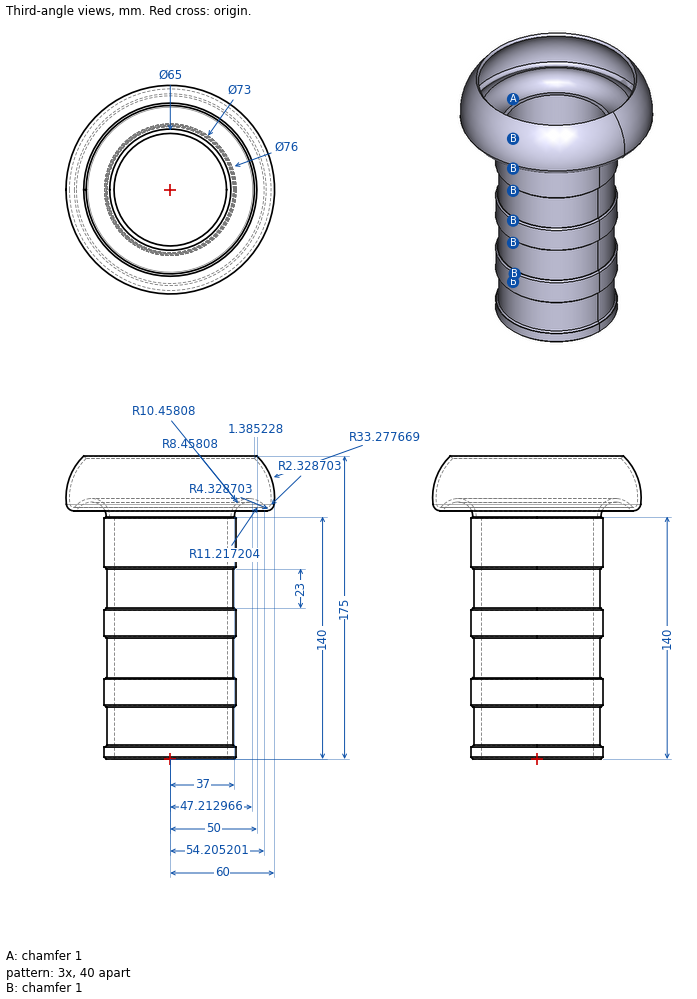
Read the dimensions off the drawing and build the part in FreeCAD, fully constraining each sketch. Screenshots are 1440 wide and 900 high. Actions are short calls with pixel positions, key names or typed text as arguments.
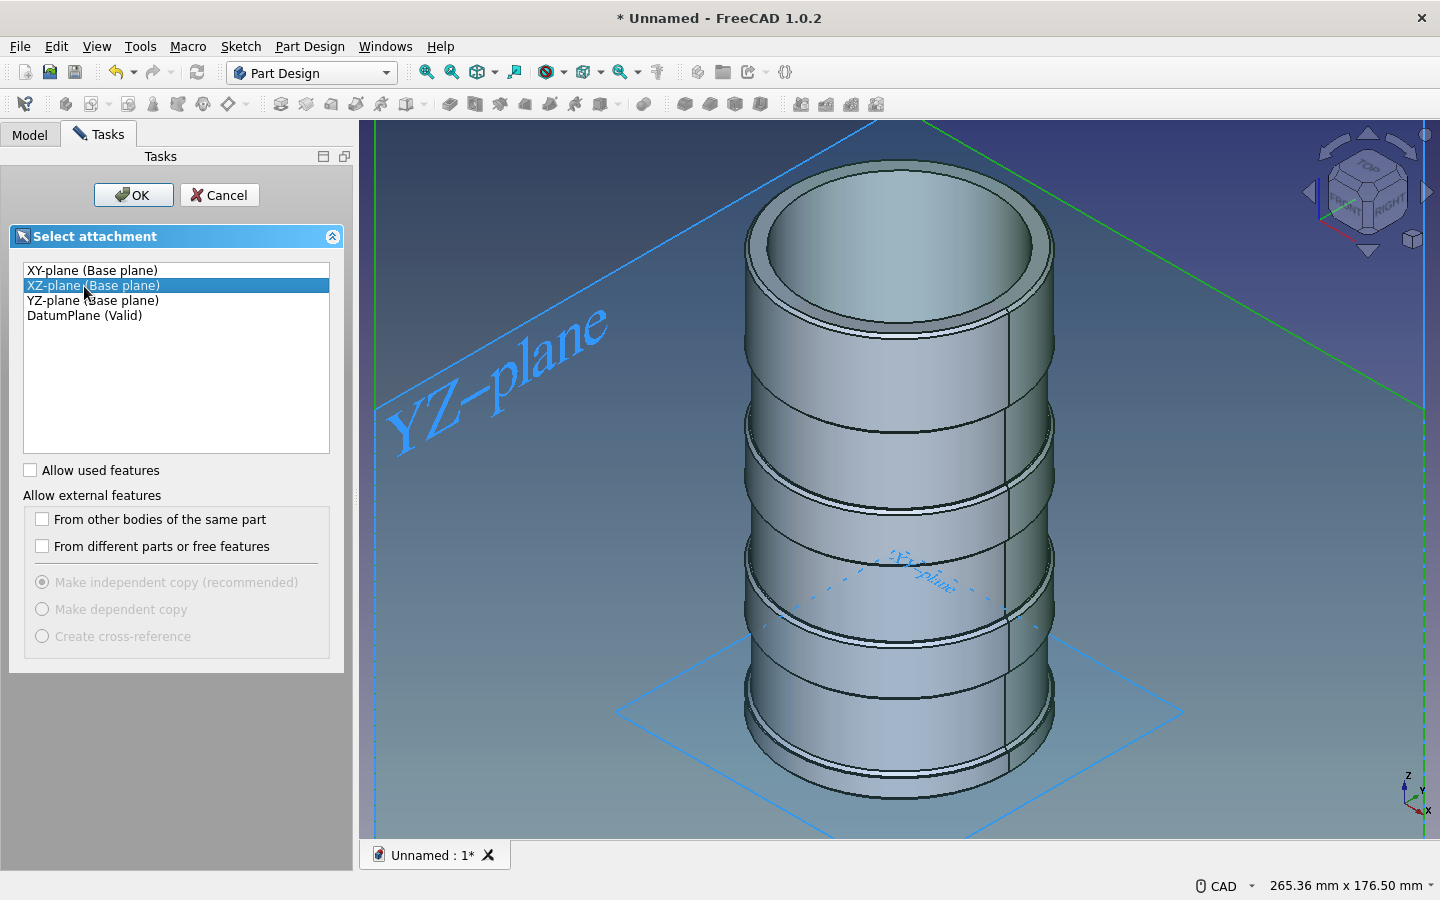
click(134, 195)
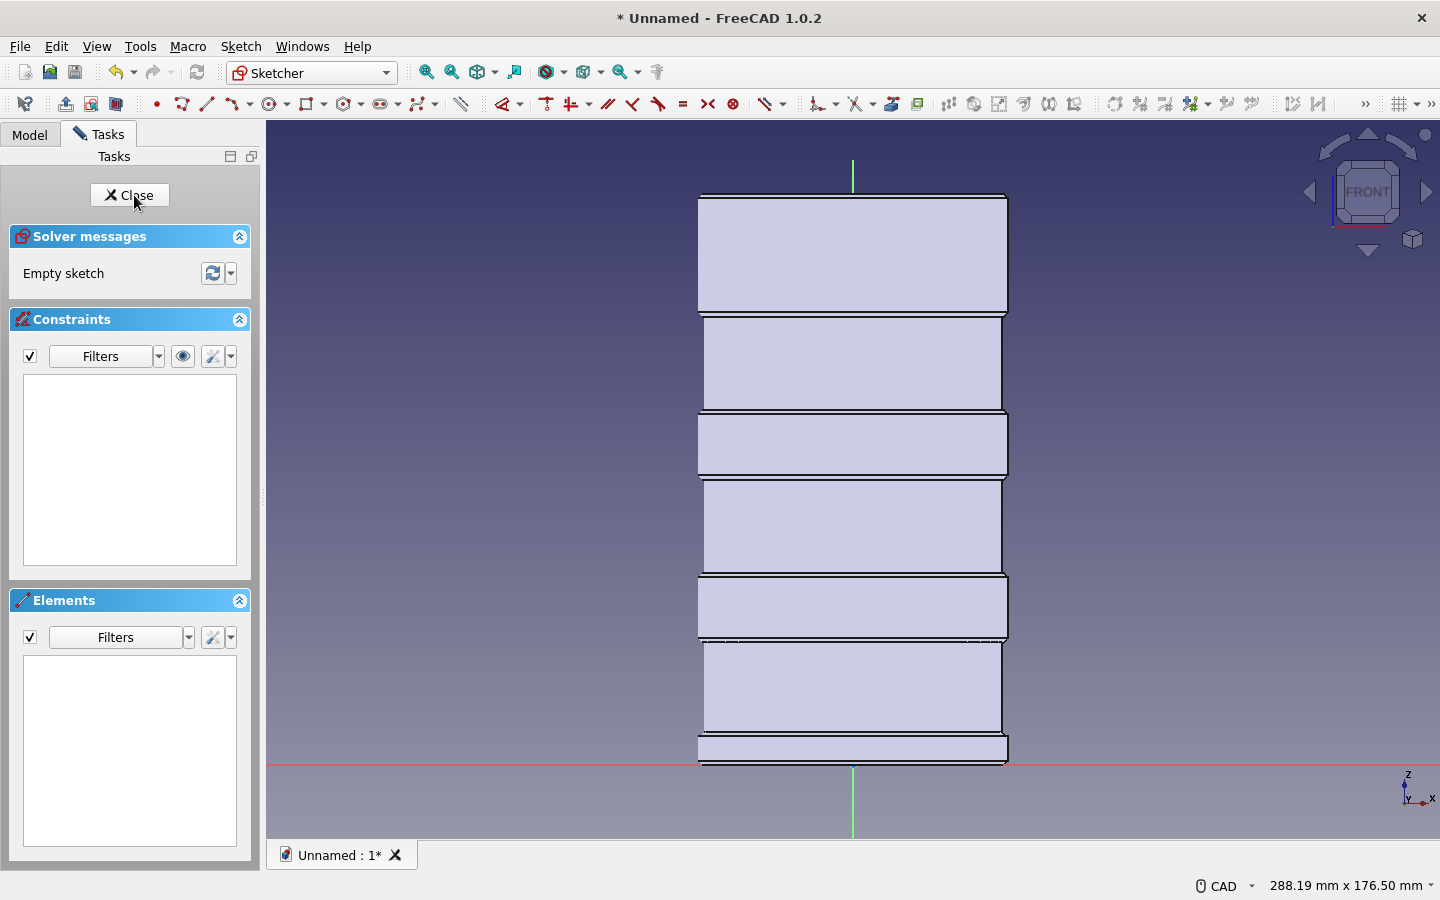
click(116, 104)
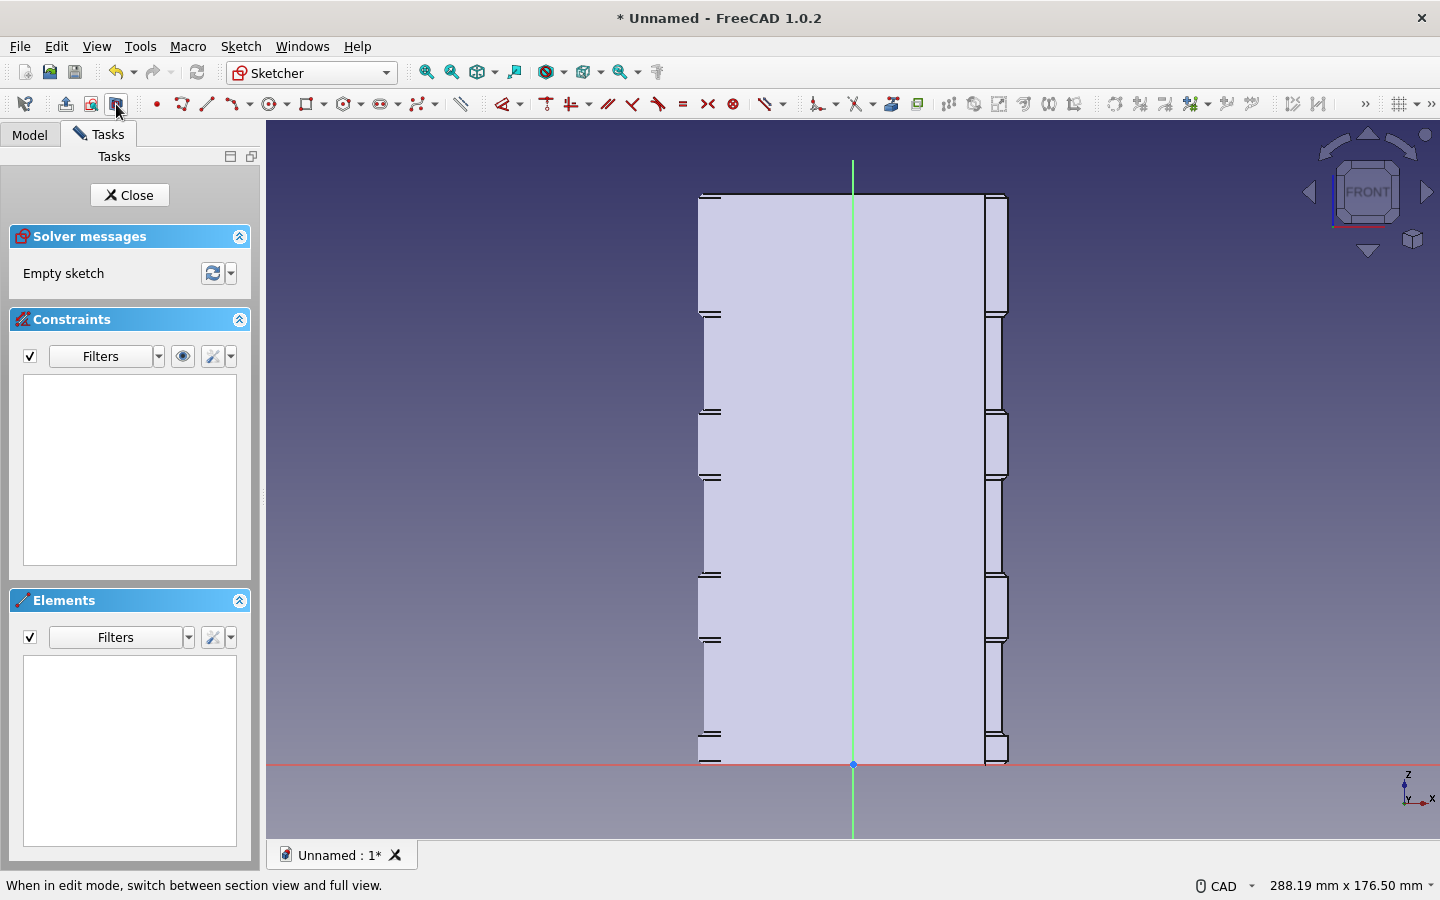
scroll(784, 480, down, 5)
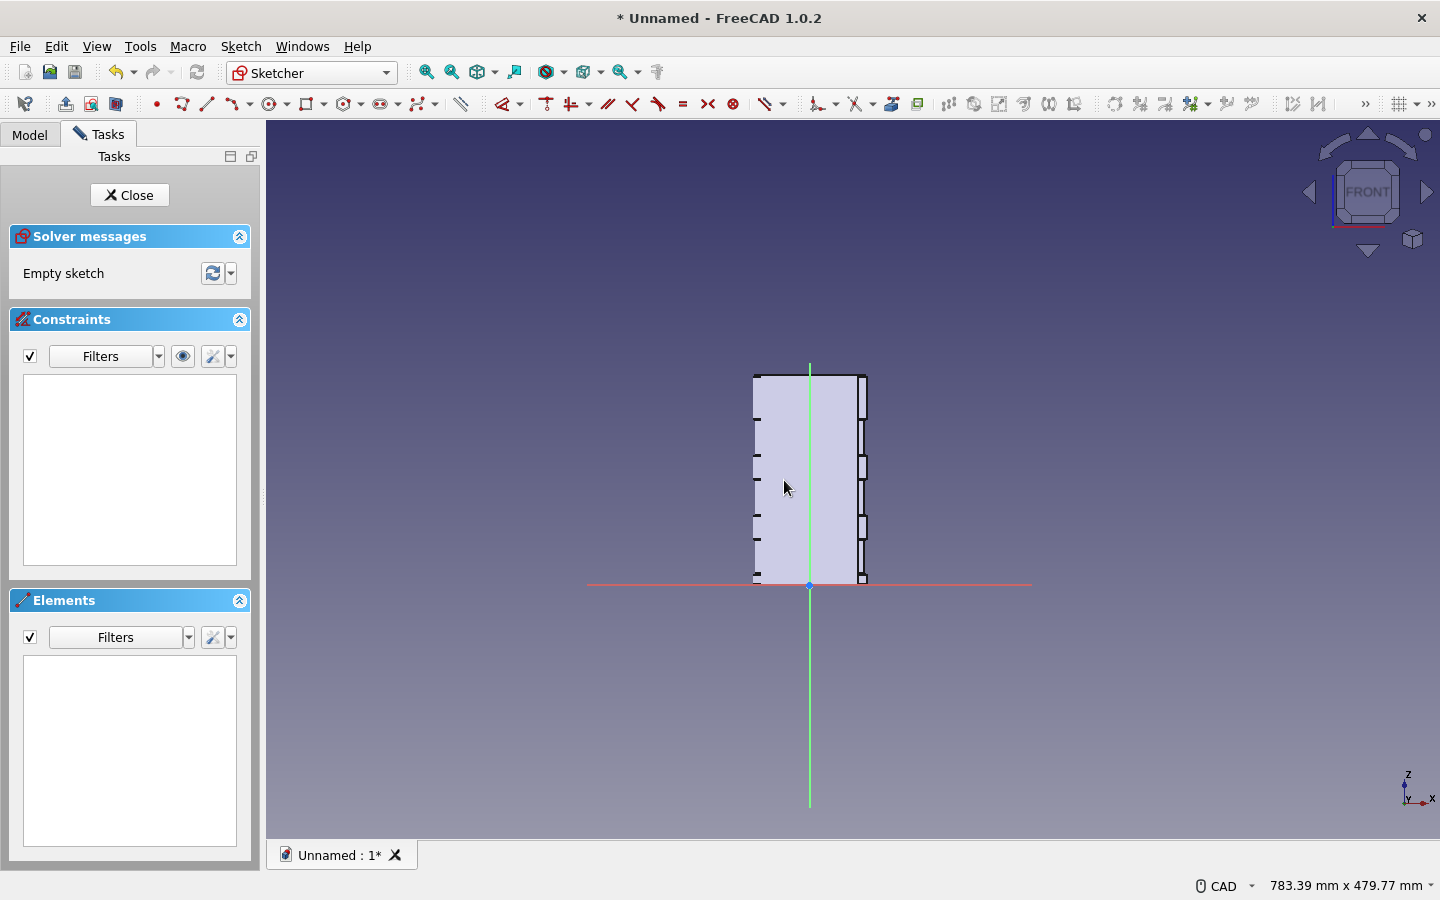
scroll(893, 333, up, 11)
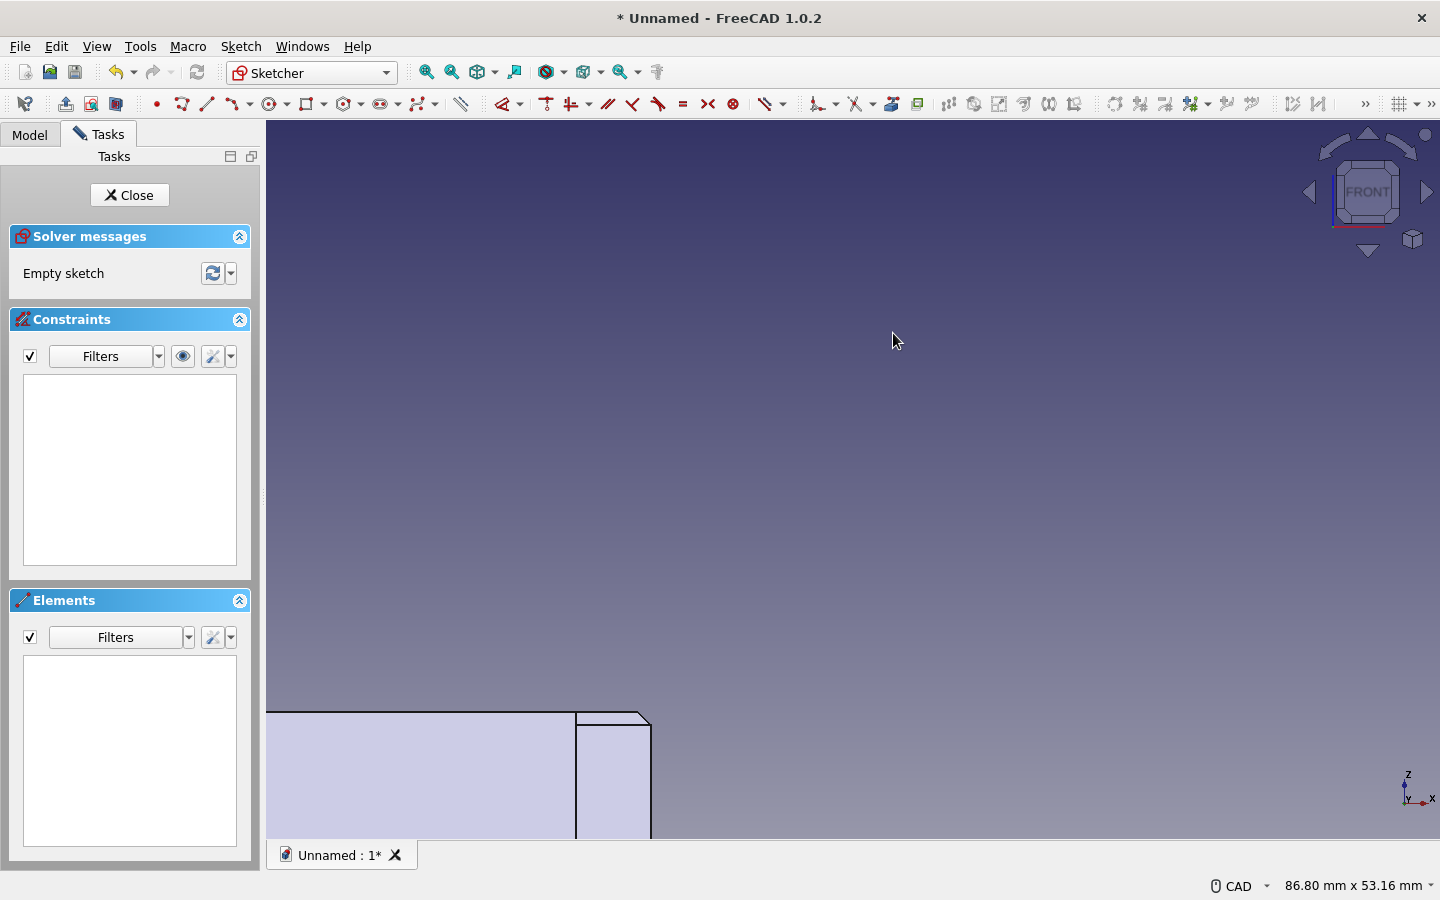
key(g)
key(l)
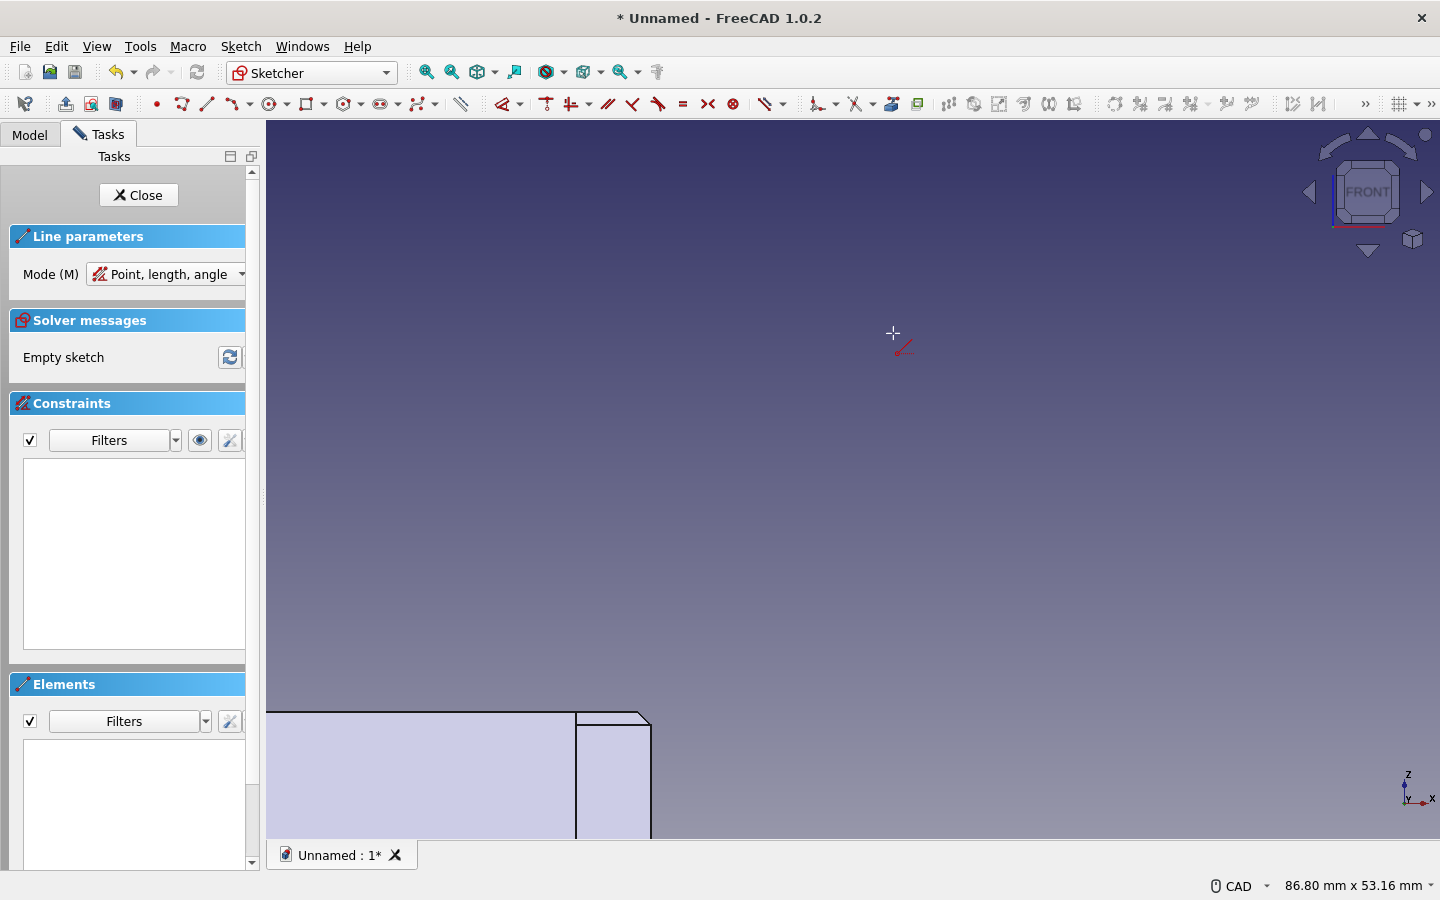
click(794, 258)
click(813, 238)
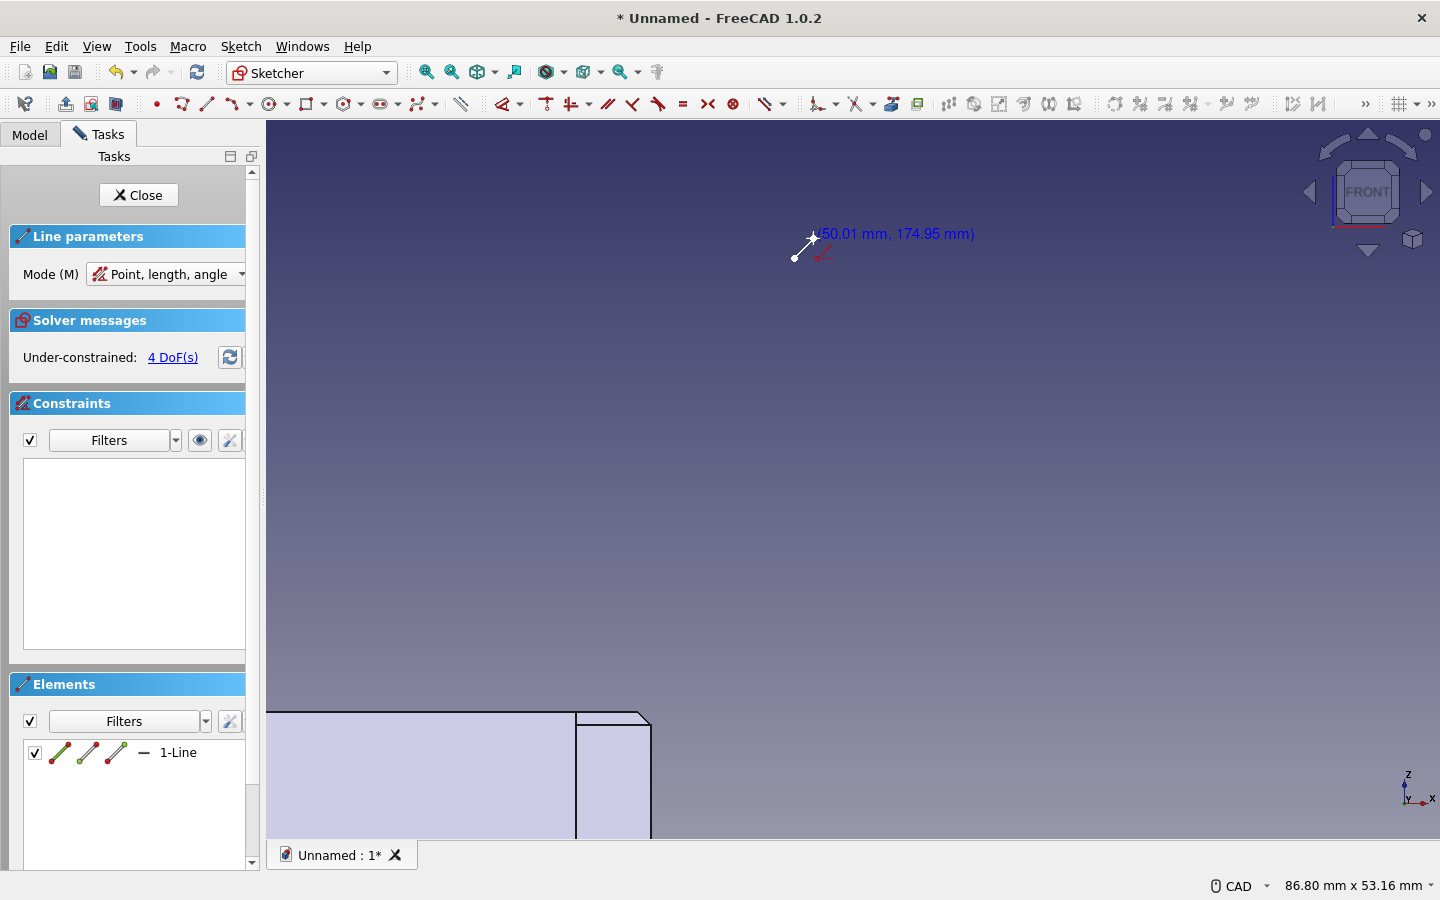
click(637, 712)
click(610, 712)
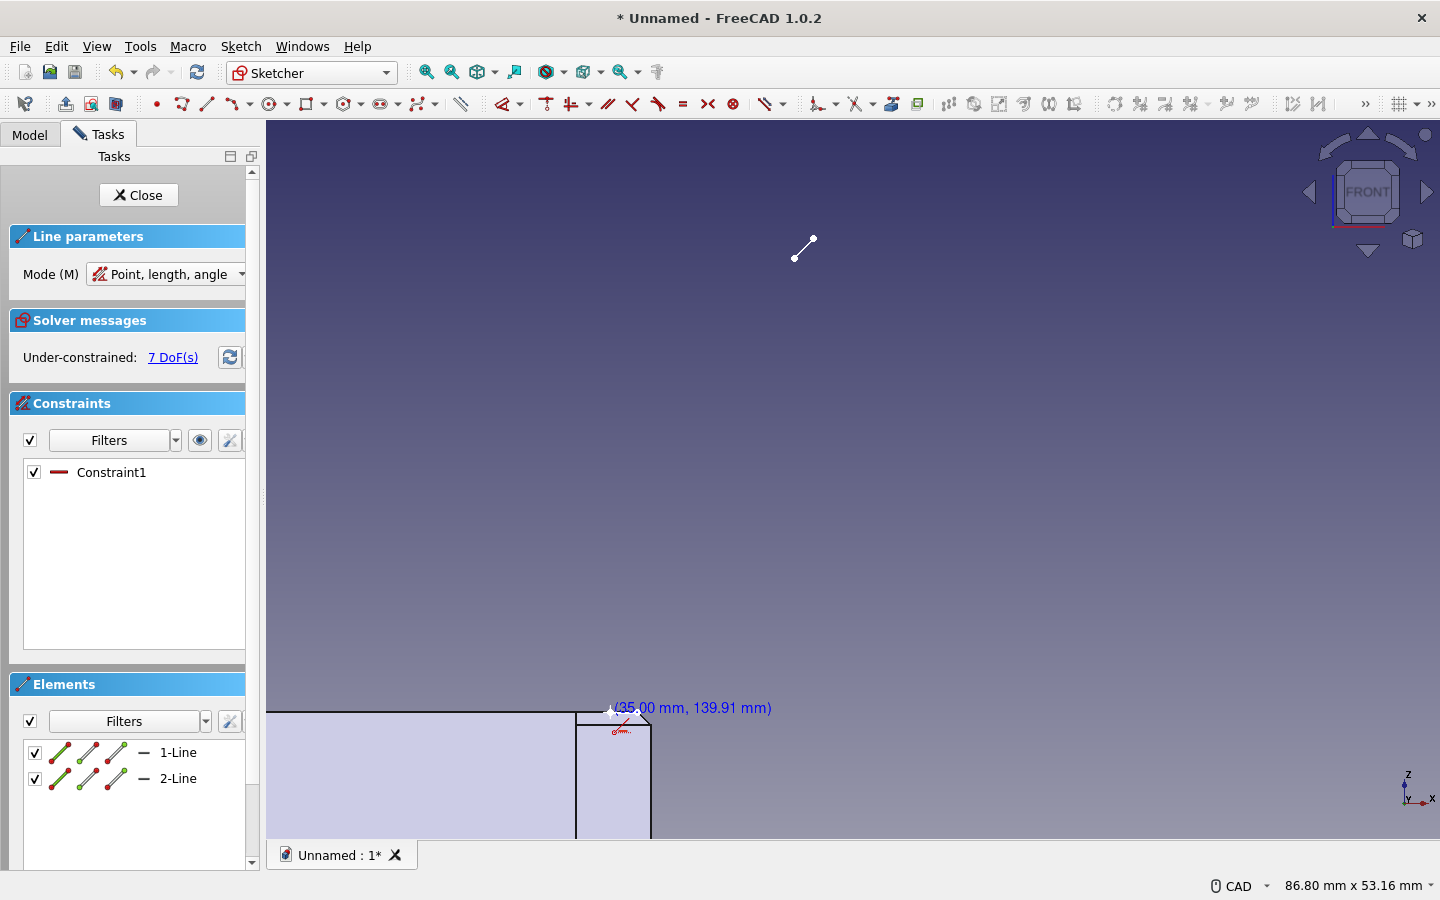
click(232, 104)